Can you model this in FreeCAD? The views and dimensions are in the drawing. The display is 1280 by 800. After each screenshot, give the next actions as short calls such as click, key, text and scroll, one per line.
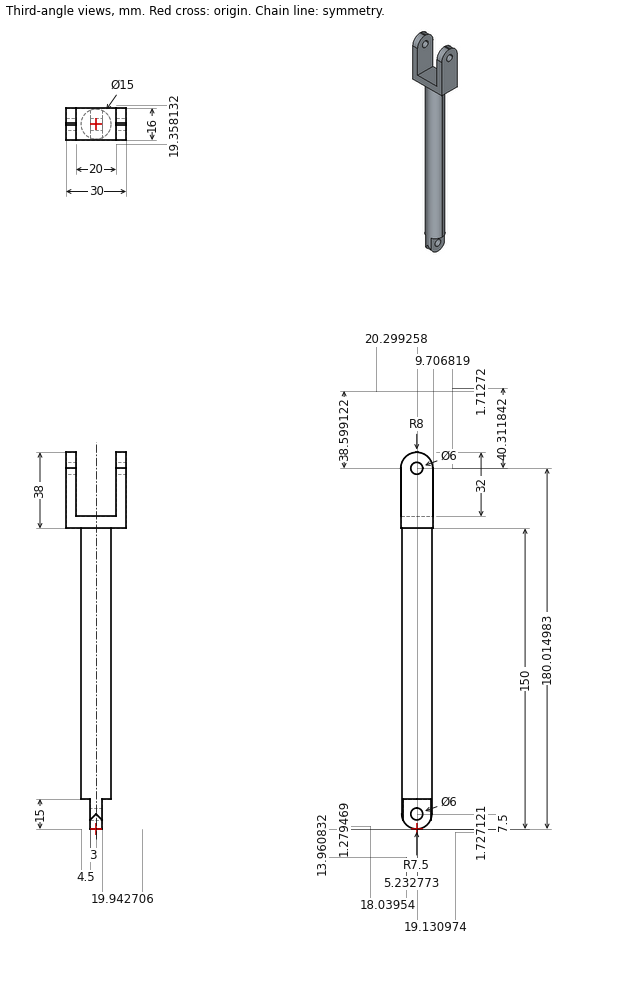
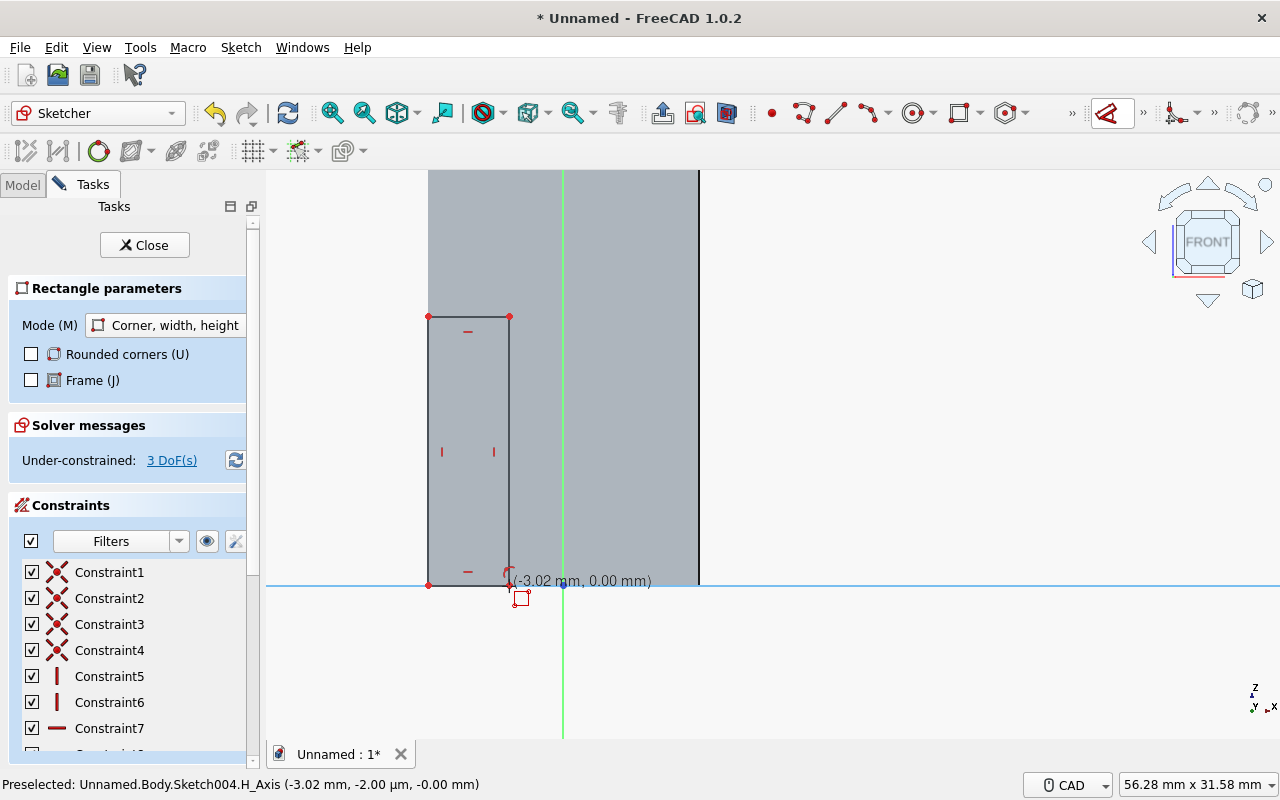
click(617, 316)
click(977, 586)
key(Escape)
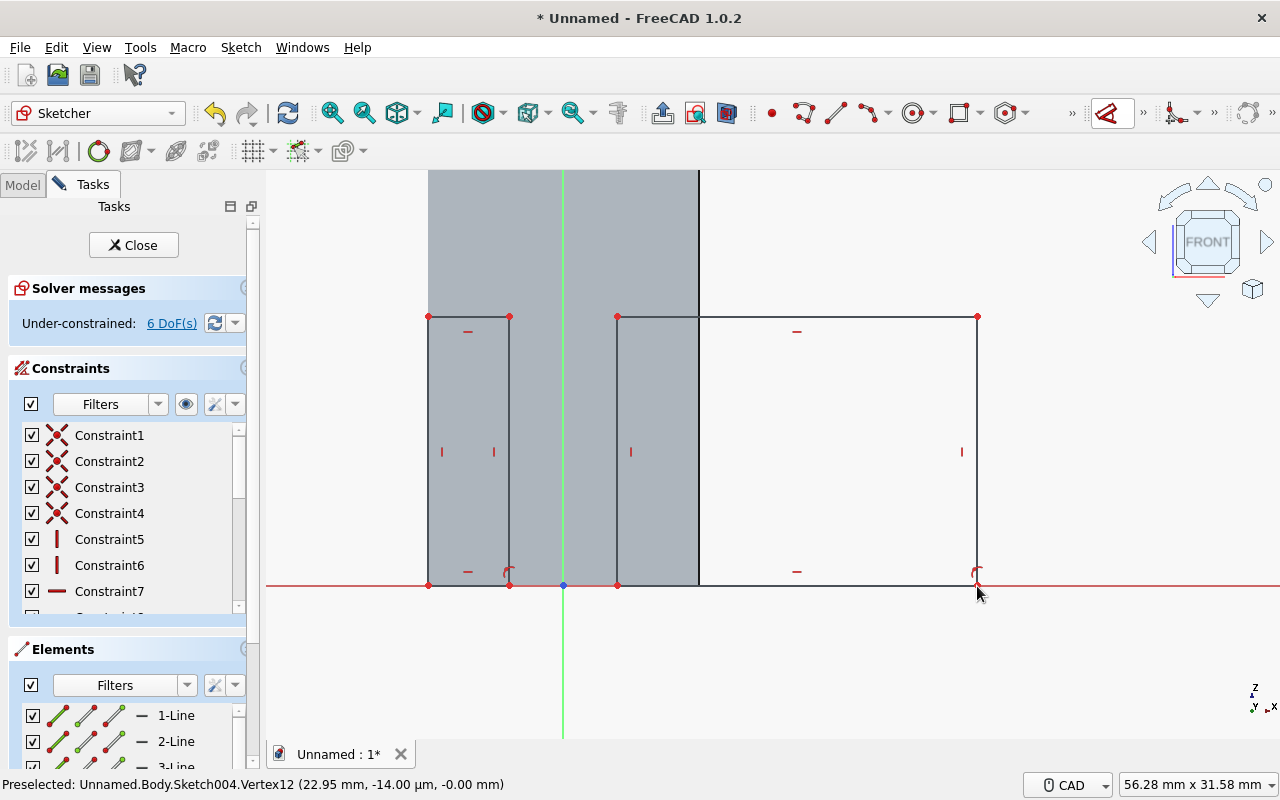
click(509, 317)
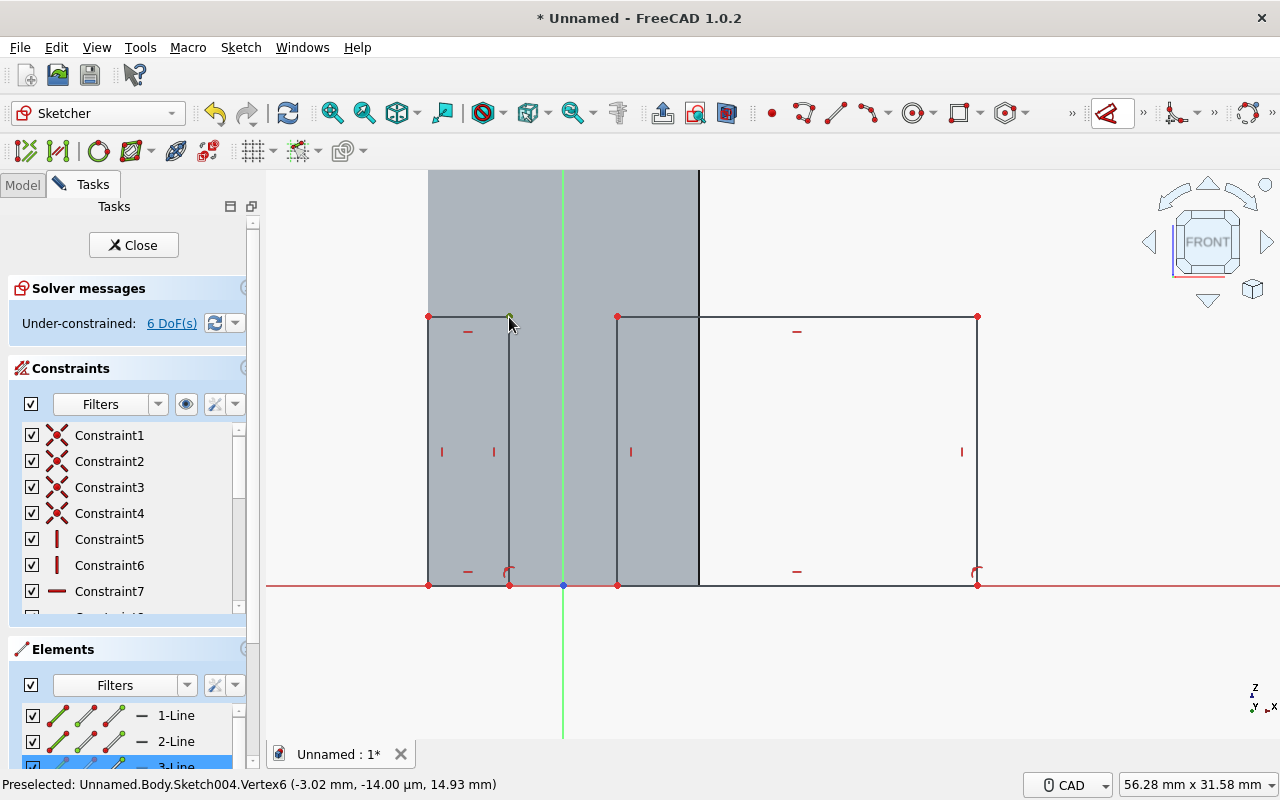
click(617, 317)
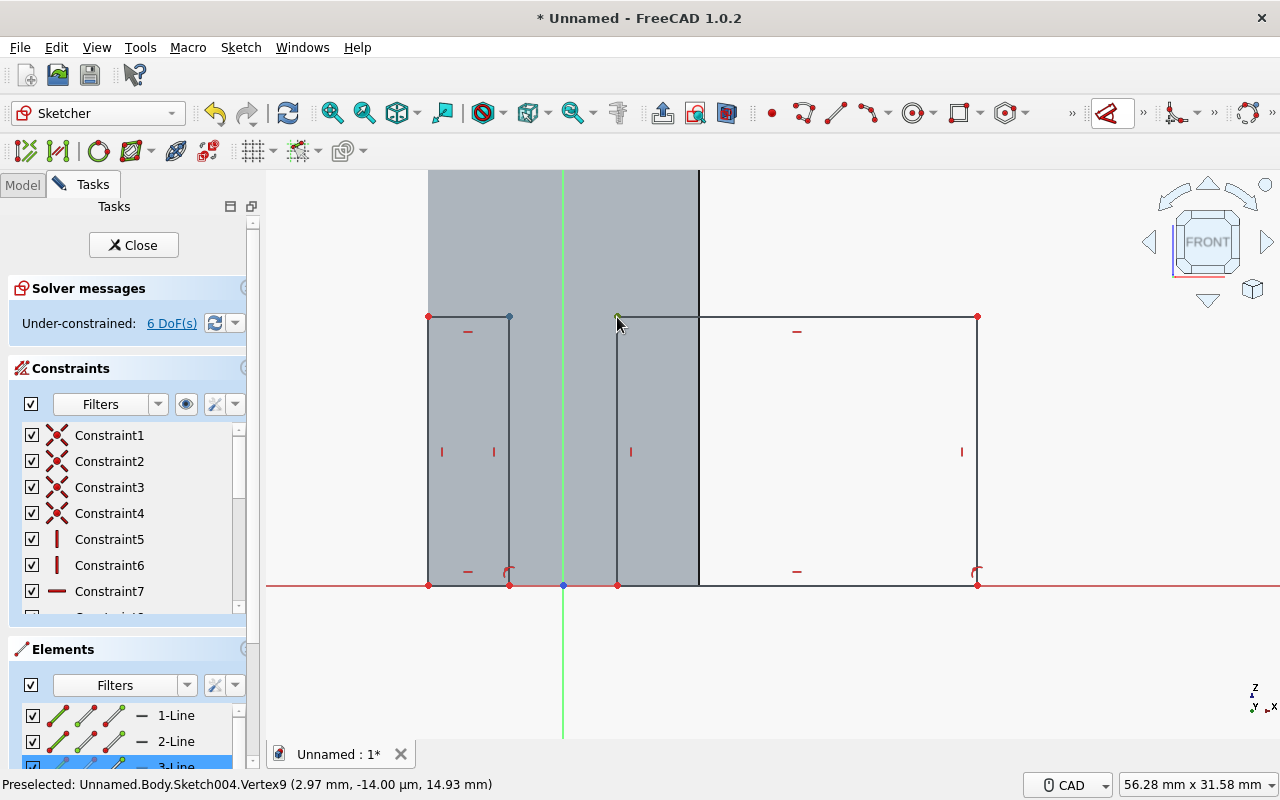
click(563, 674)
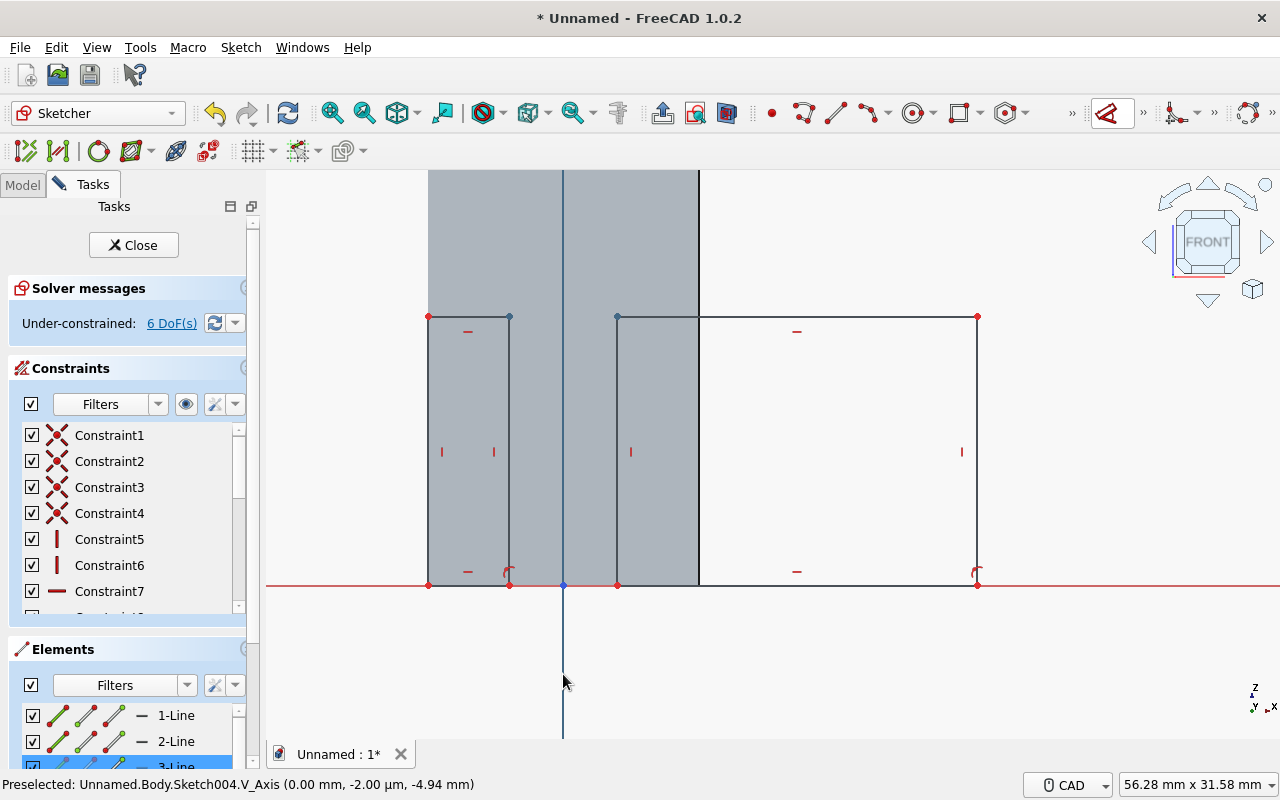
key(s)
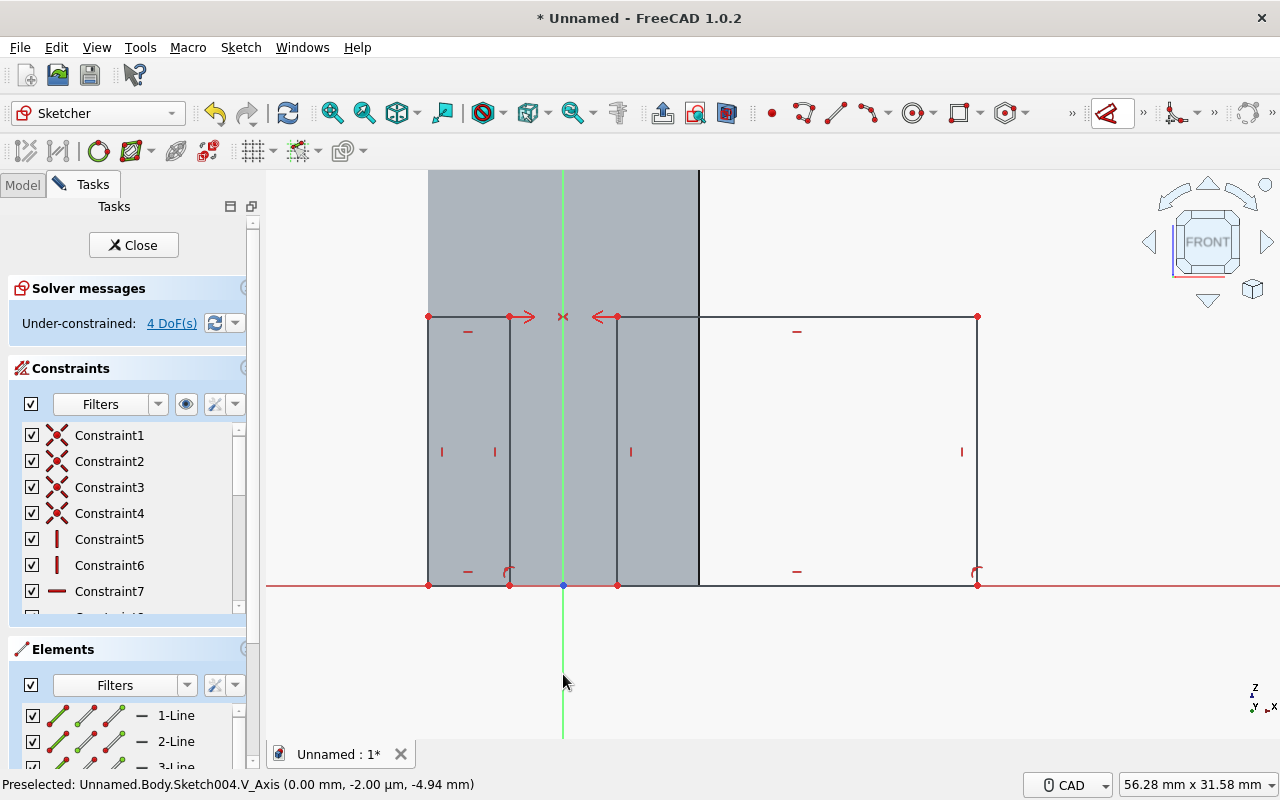
key(d)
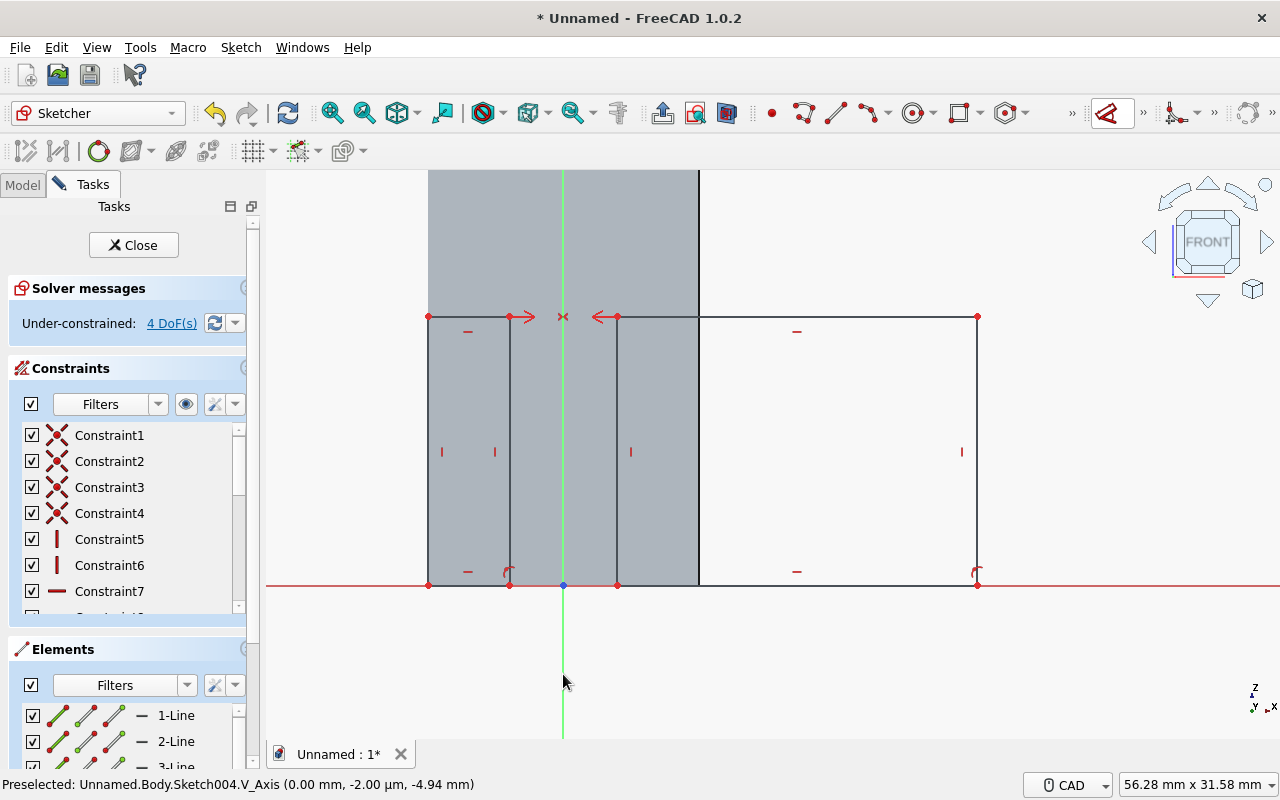
click(428, 398)
click(394, 451)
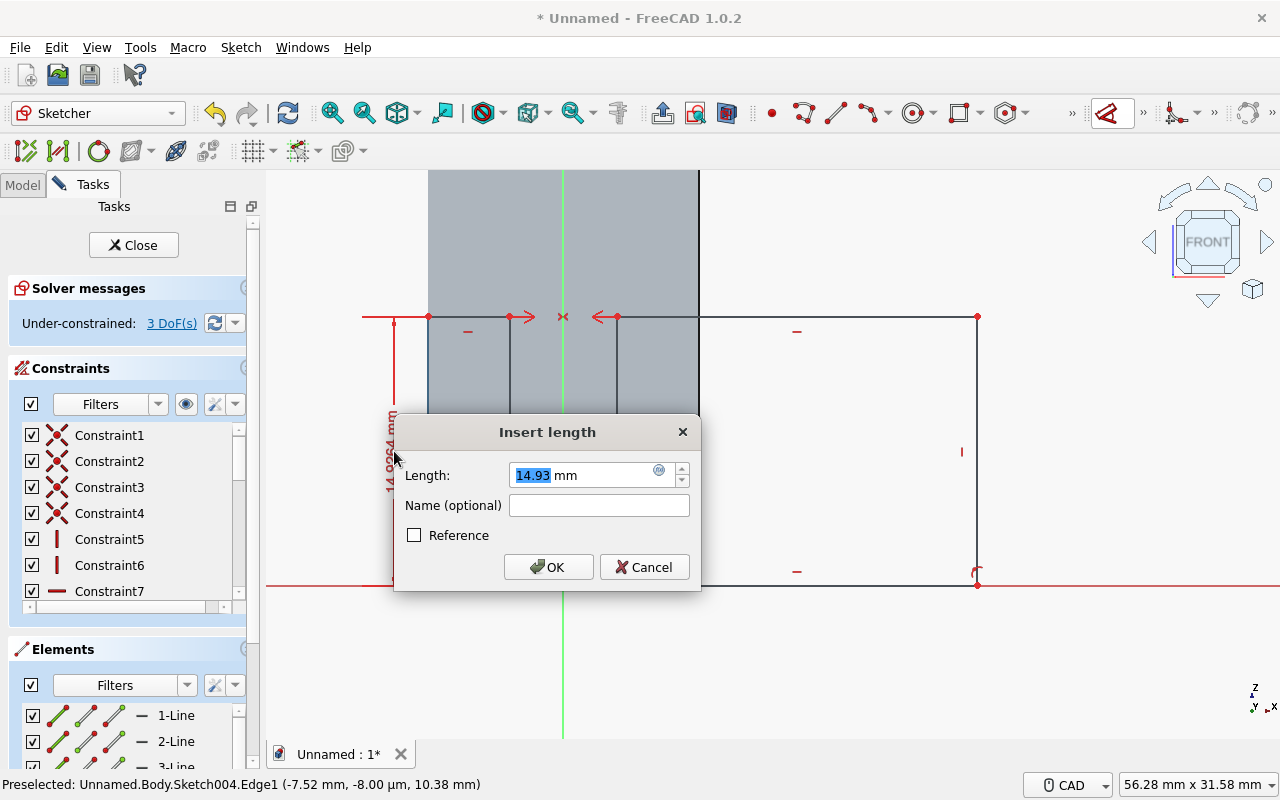
text(15)
key(Return)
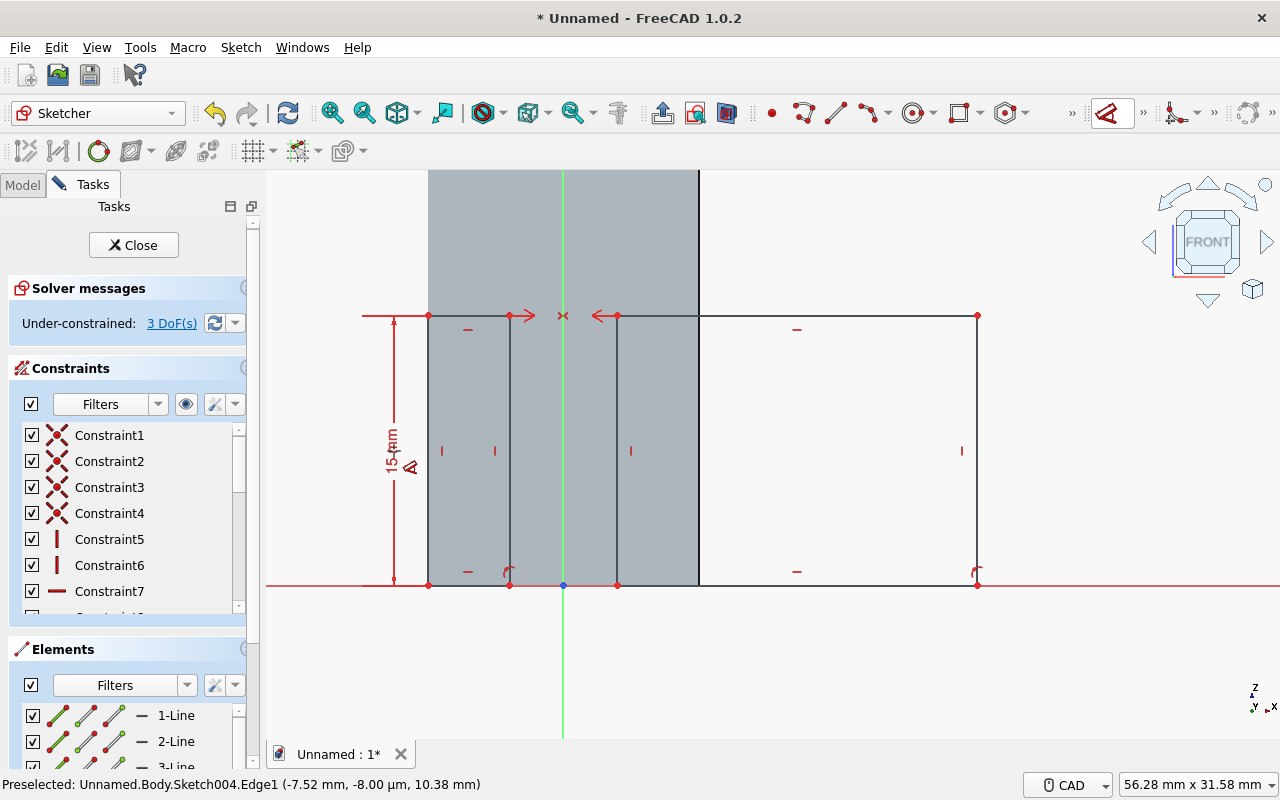
click(510, 586)
click(537, 620)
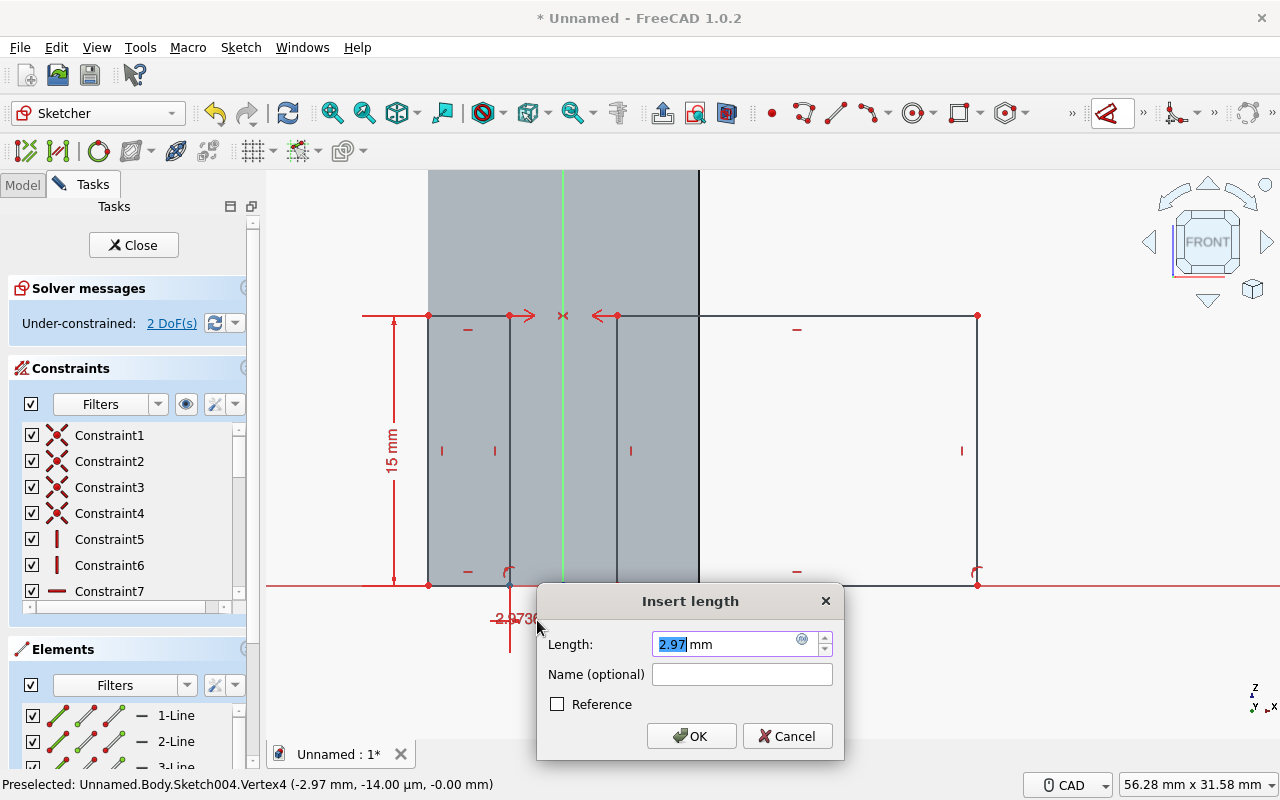
text(3)
key(Return)